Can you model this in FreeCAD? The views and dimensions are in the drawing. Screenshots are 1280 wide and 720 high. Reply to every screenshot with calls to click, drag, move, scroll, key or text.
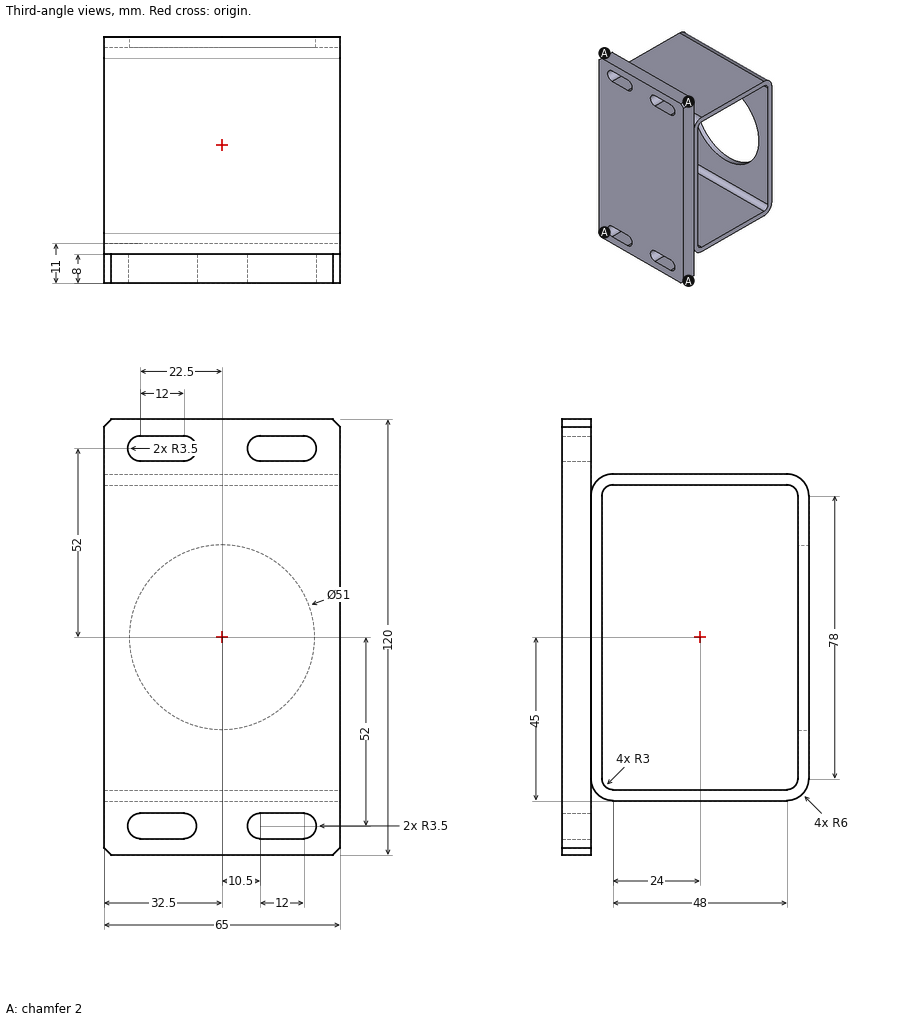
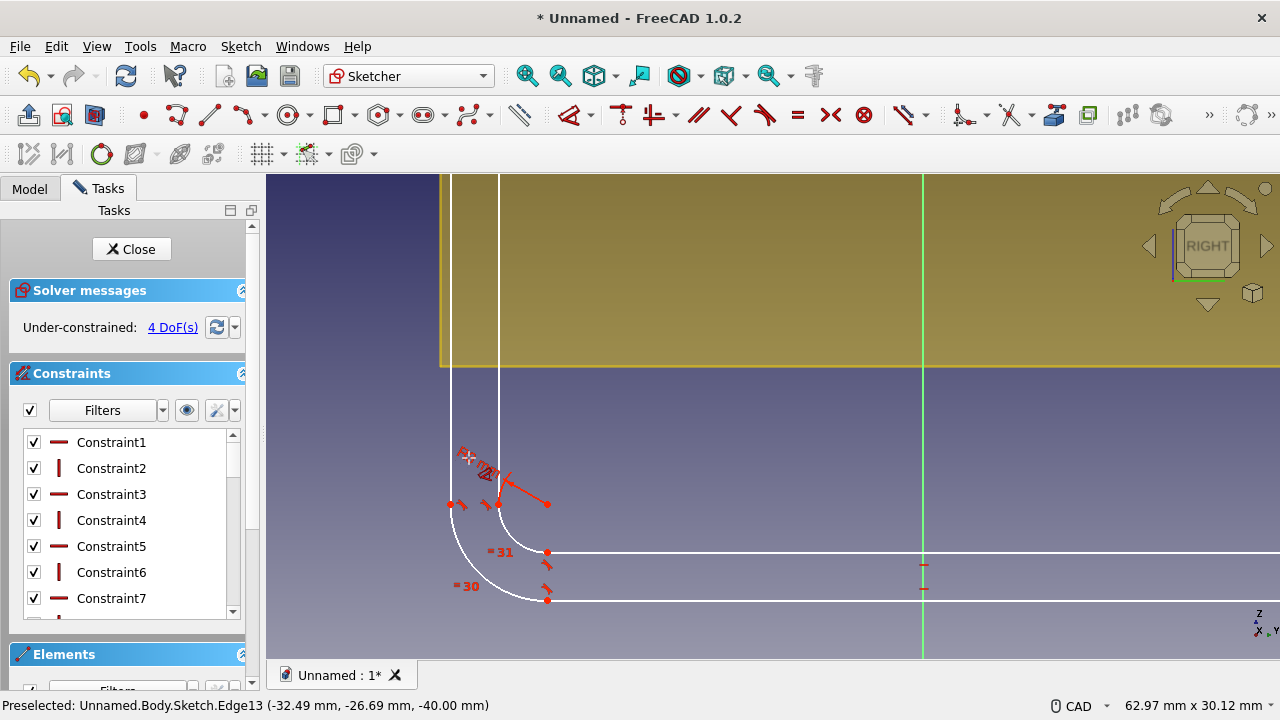
scroll(649, 551, down, 8)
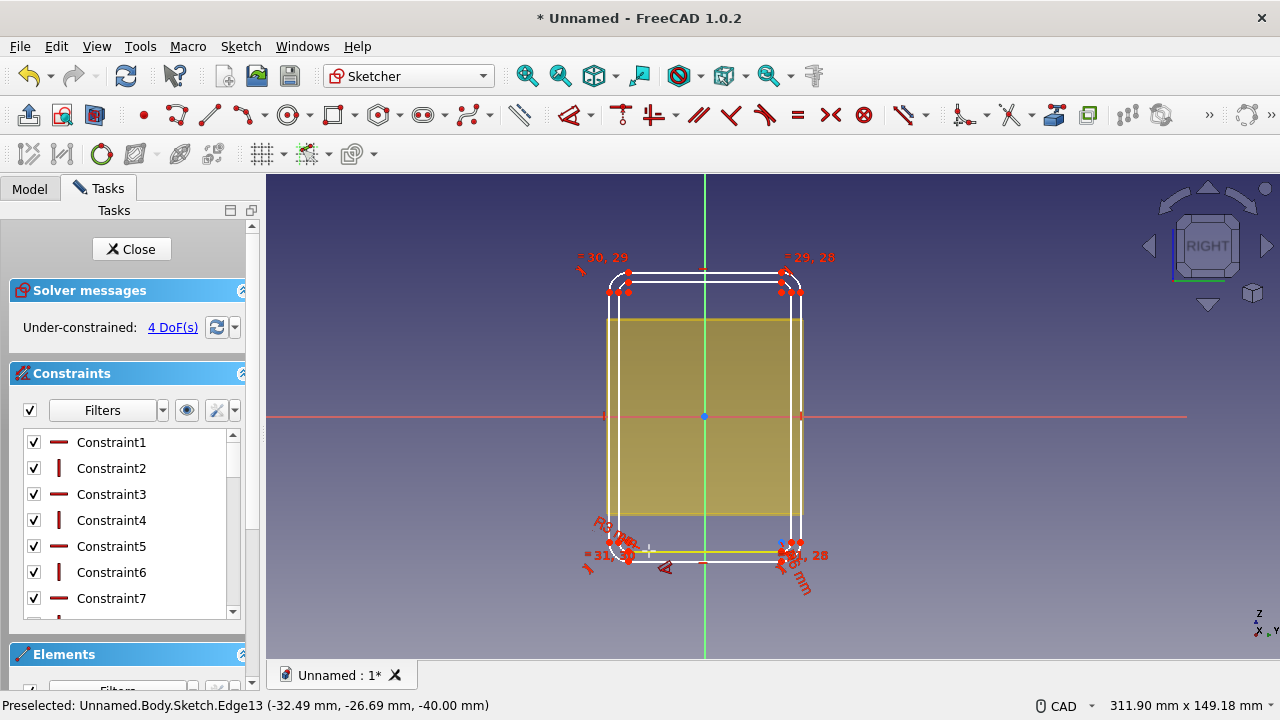
scroll(675, 562, up, 2)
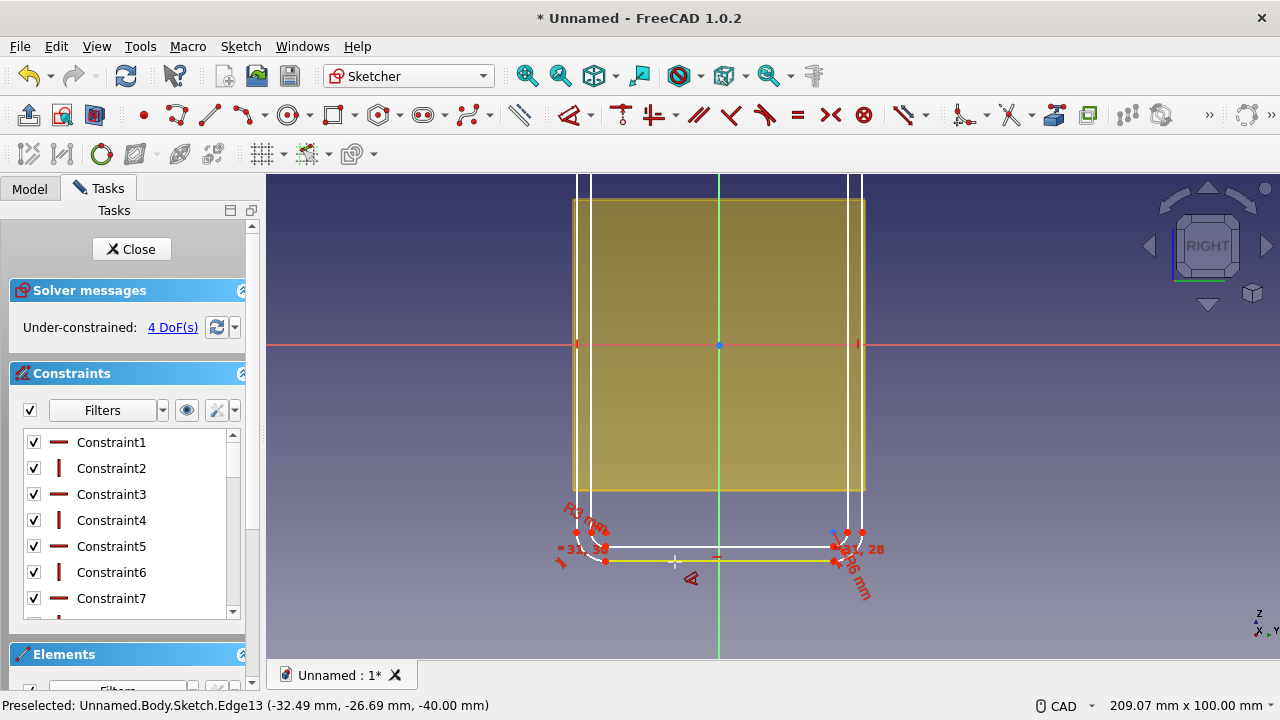
click(674, 561)
click(667, 595)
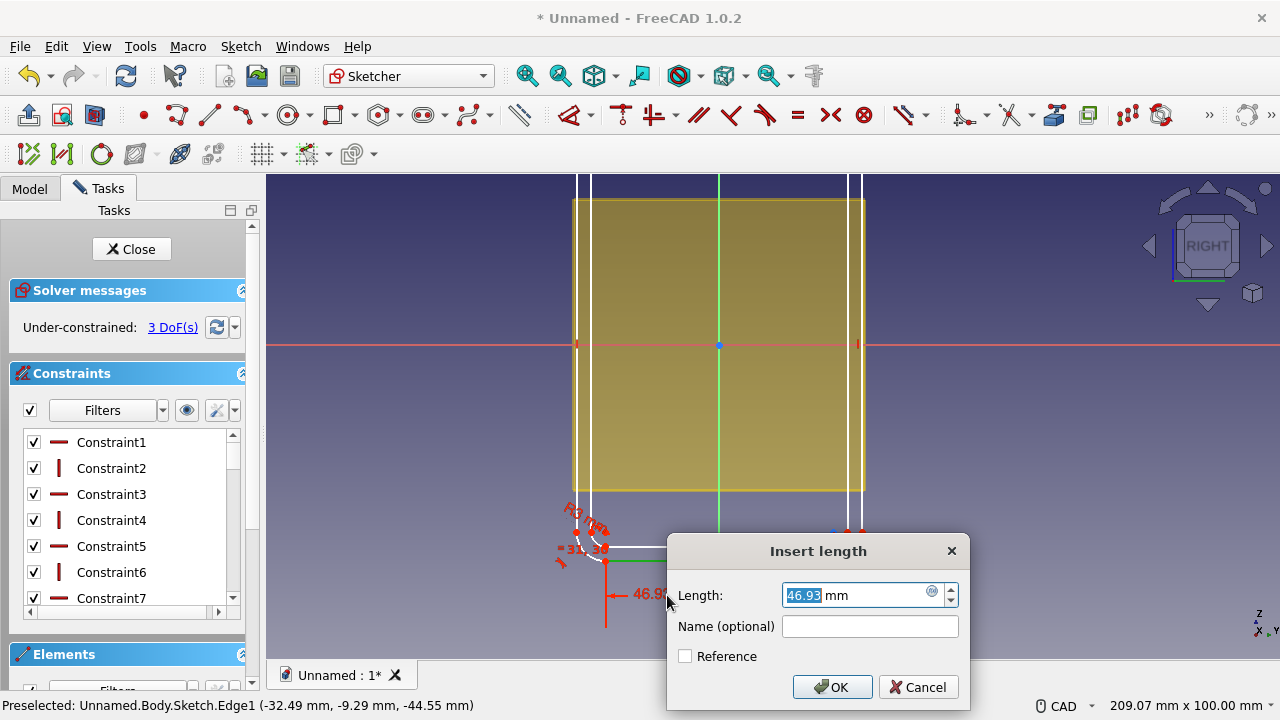
text(48)
key(Return)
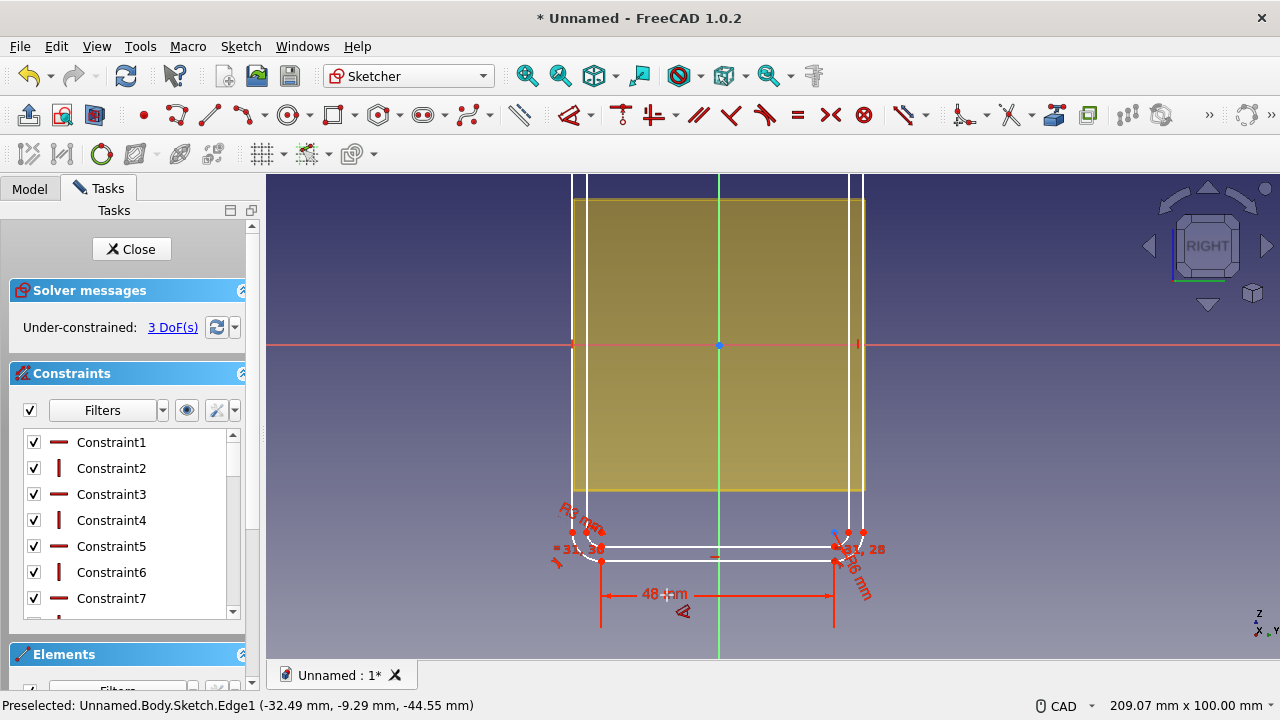
click(863, 420)
click(897, 367)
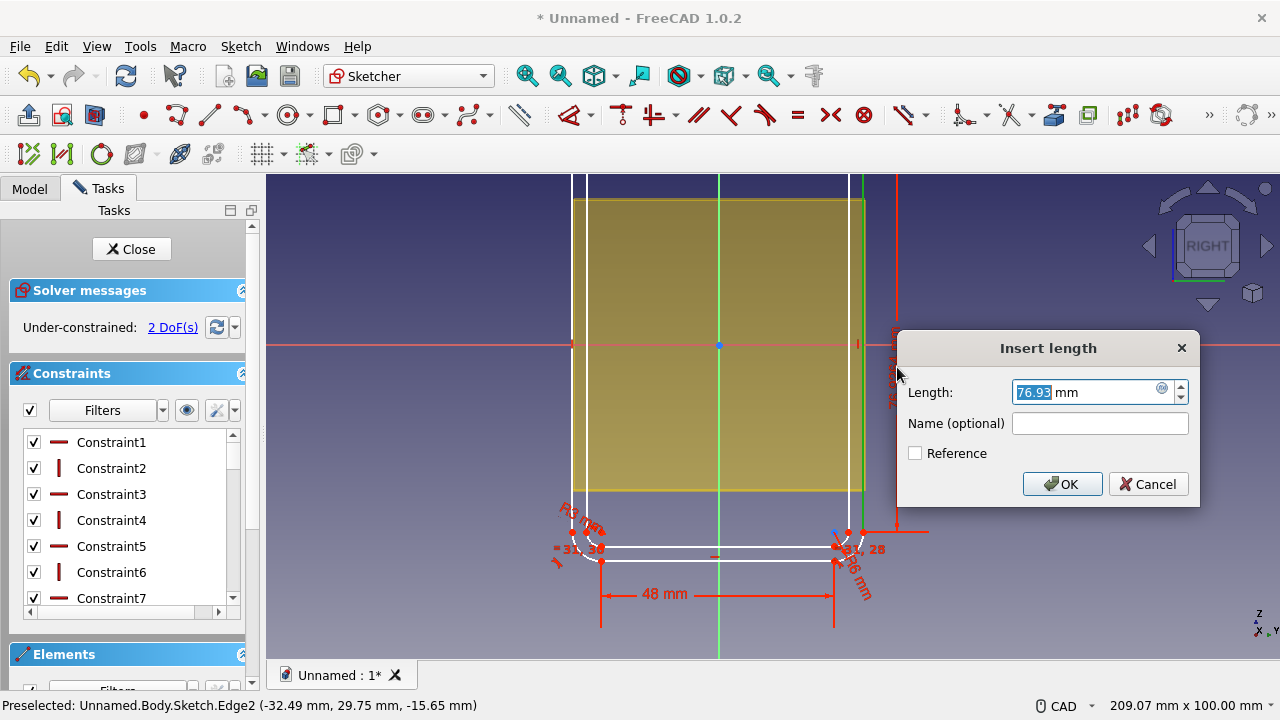
text(78)
key(Return)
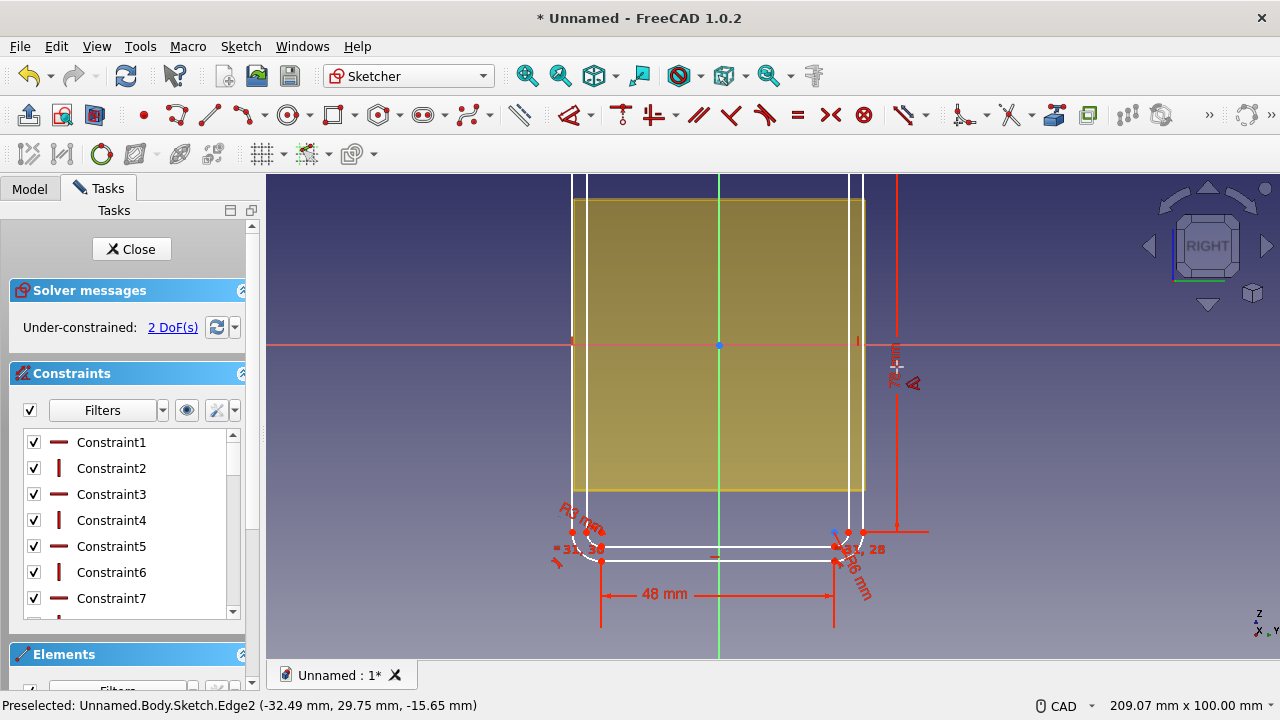
click(601, 561)
click(660, 311)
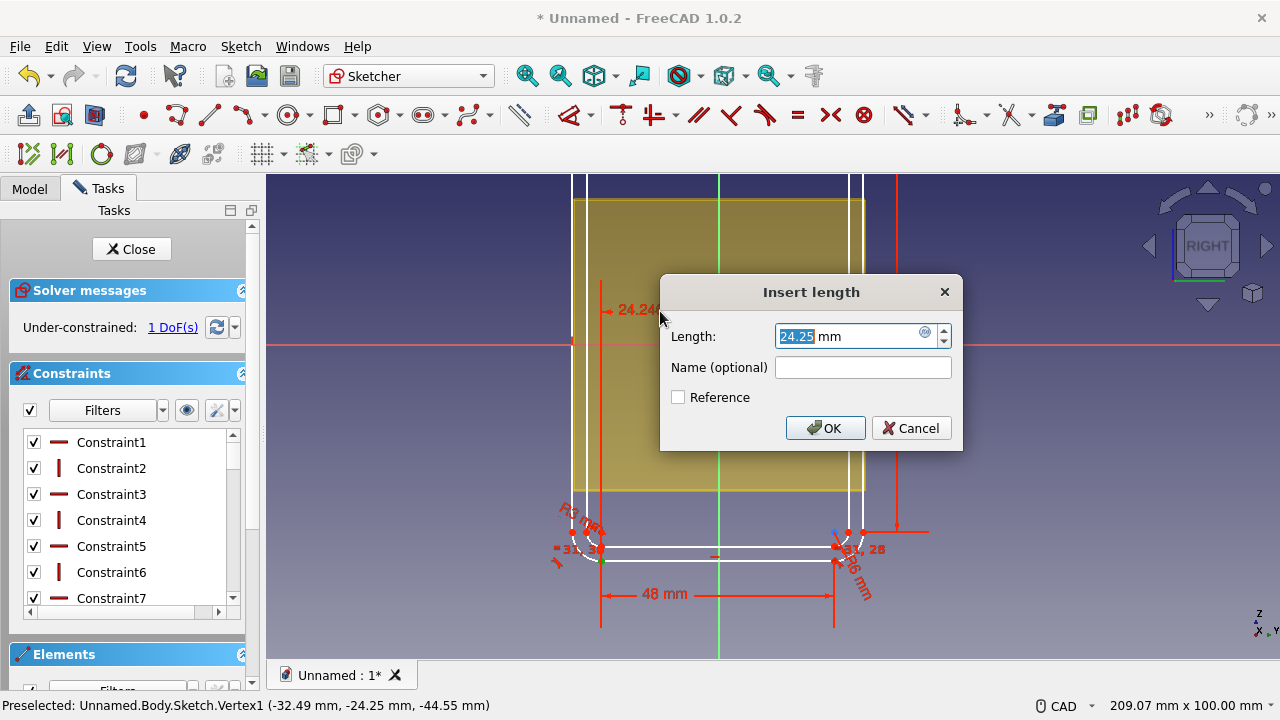
text(24)
key(Return)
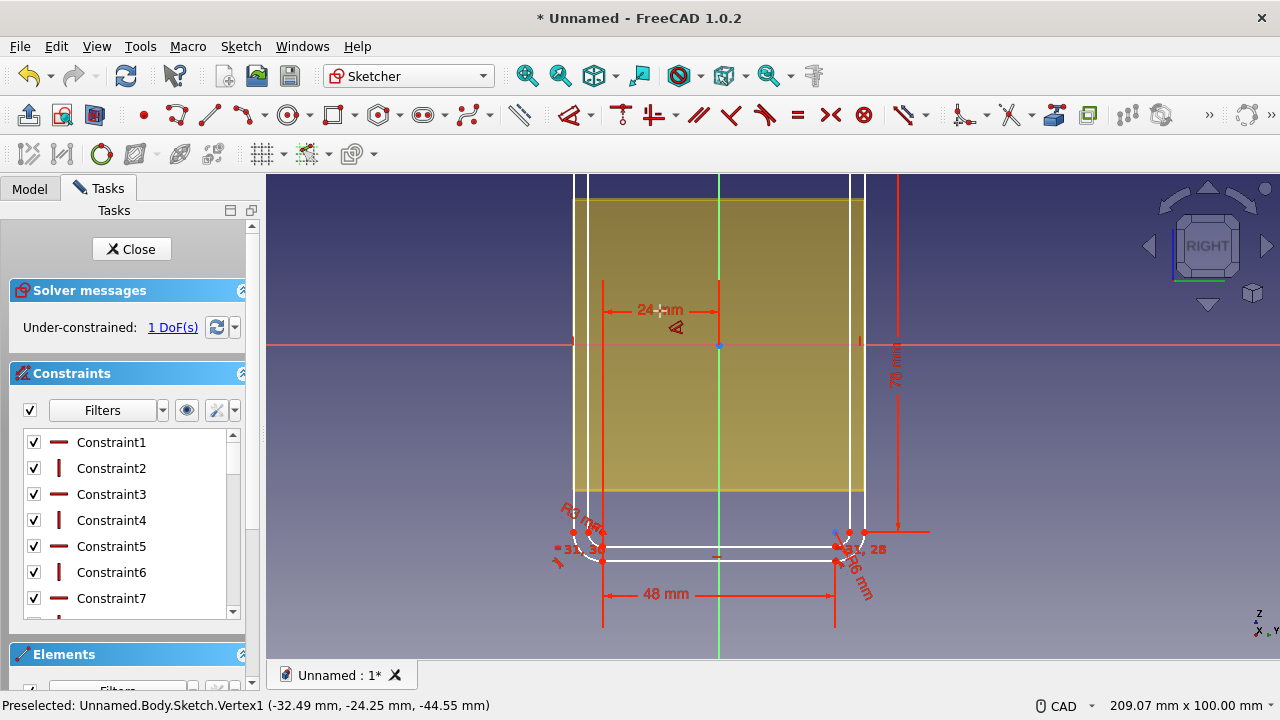
click(603, 561)
click(753, 453)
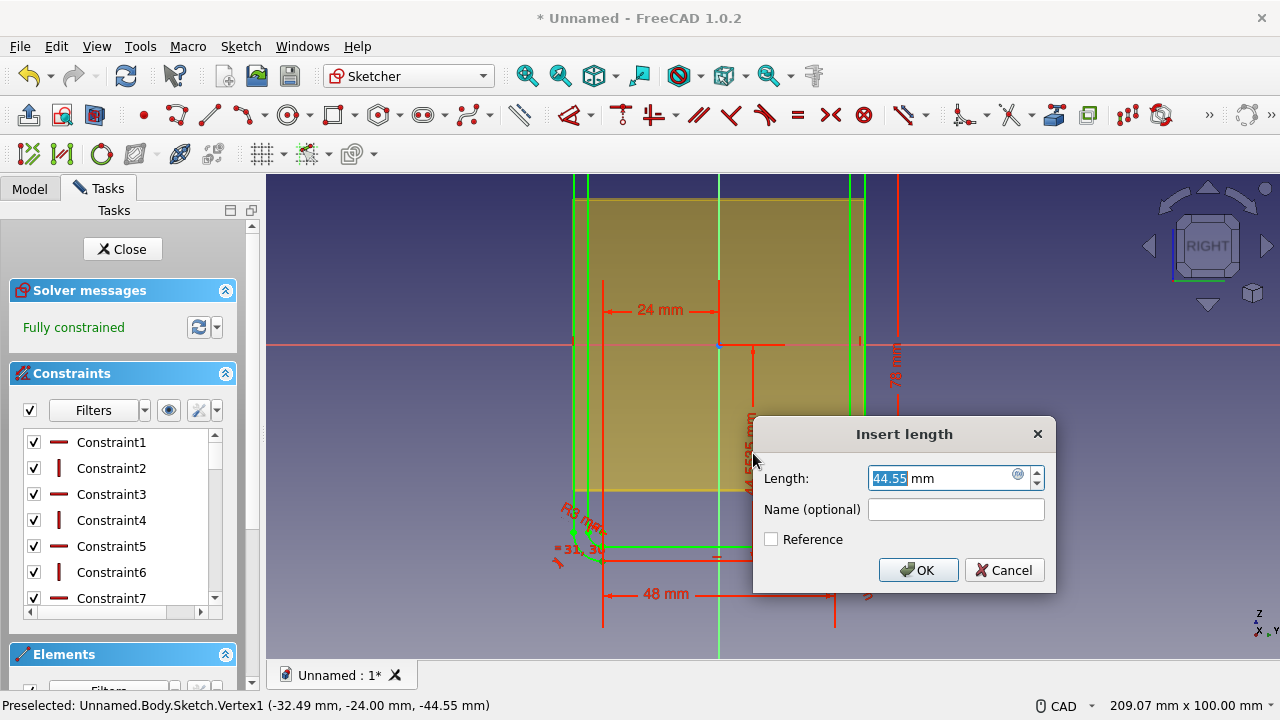
text(45)
key(Return)
key(Escape)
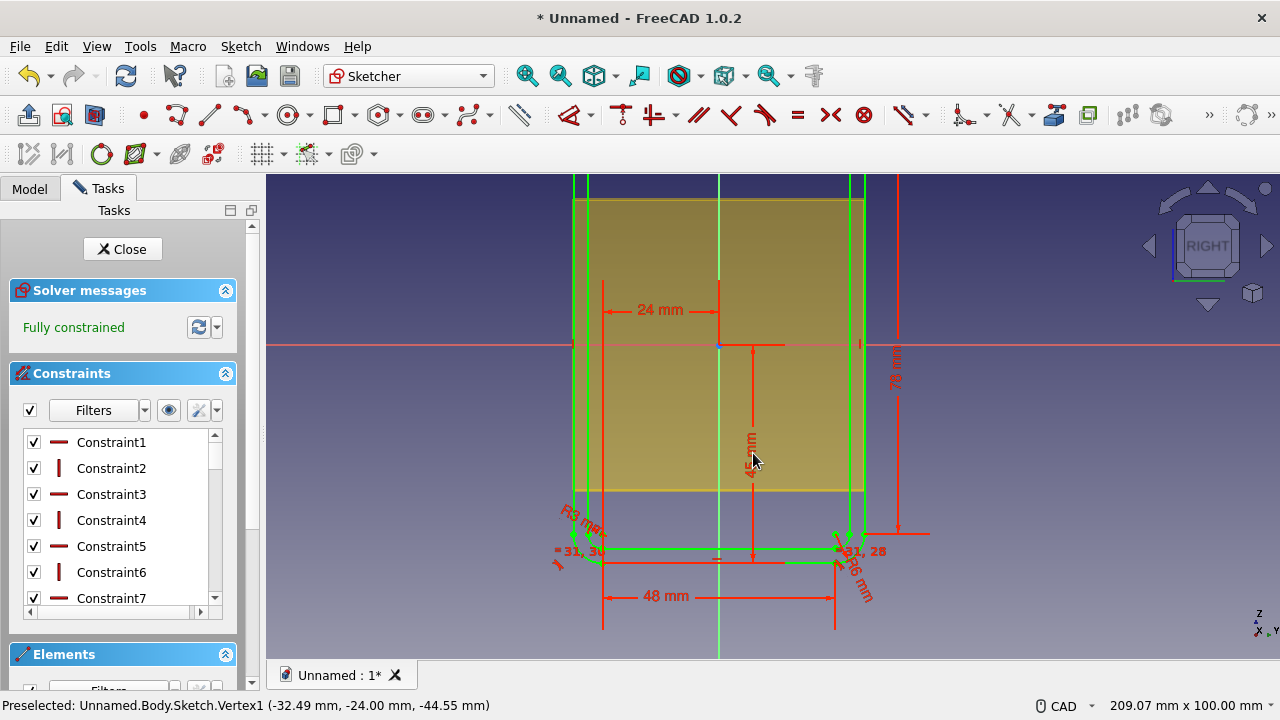
click(123, 249)